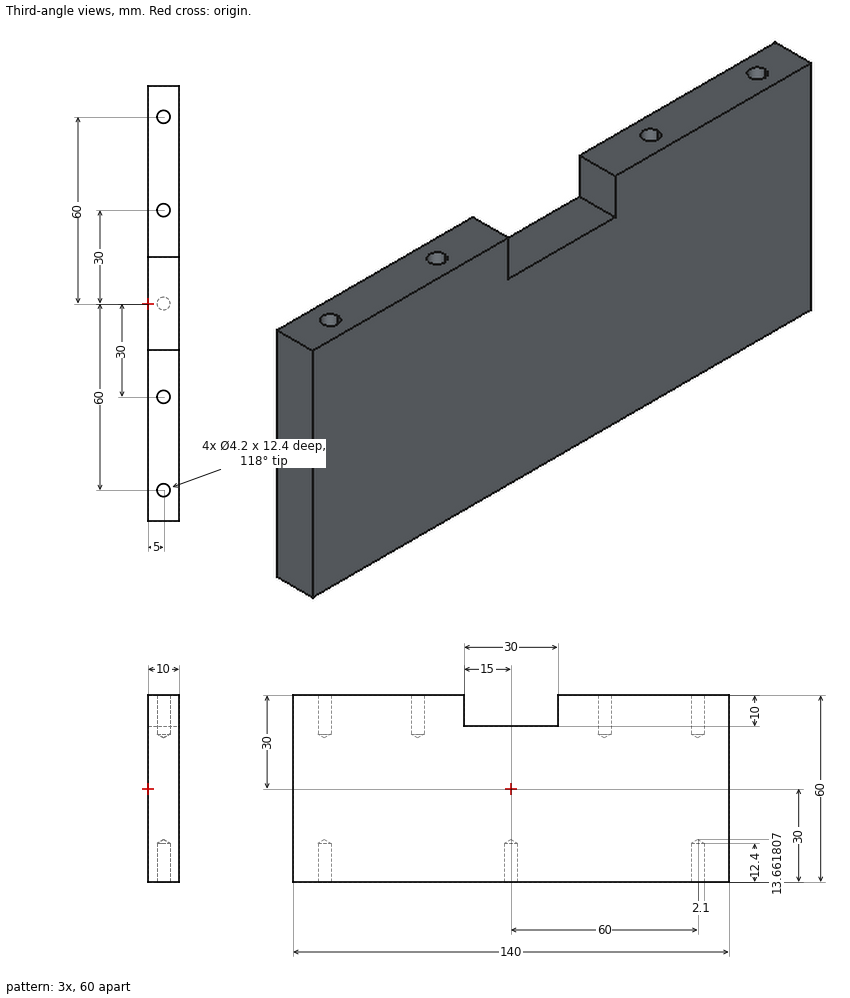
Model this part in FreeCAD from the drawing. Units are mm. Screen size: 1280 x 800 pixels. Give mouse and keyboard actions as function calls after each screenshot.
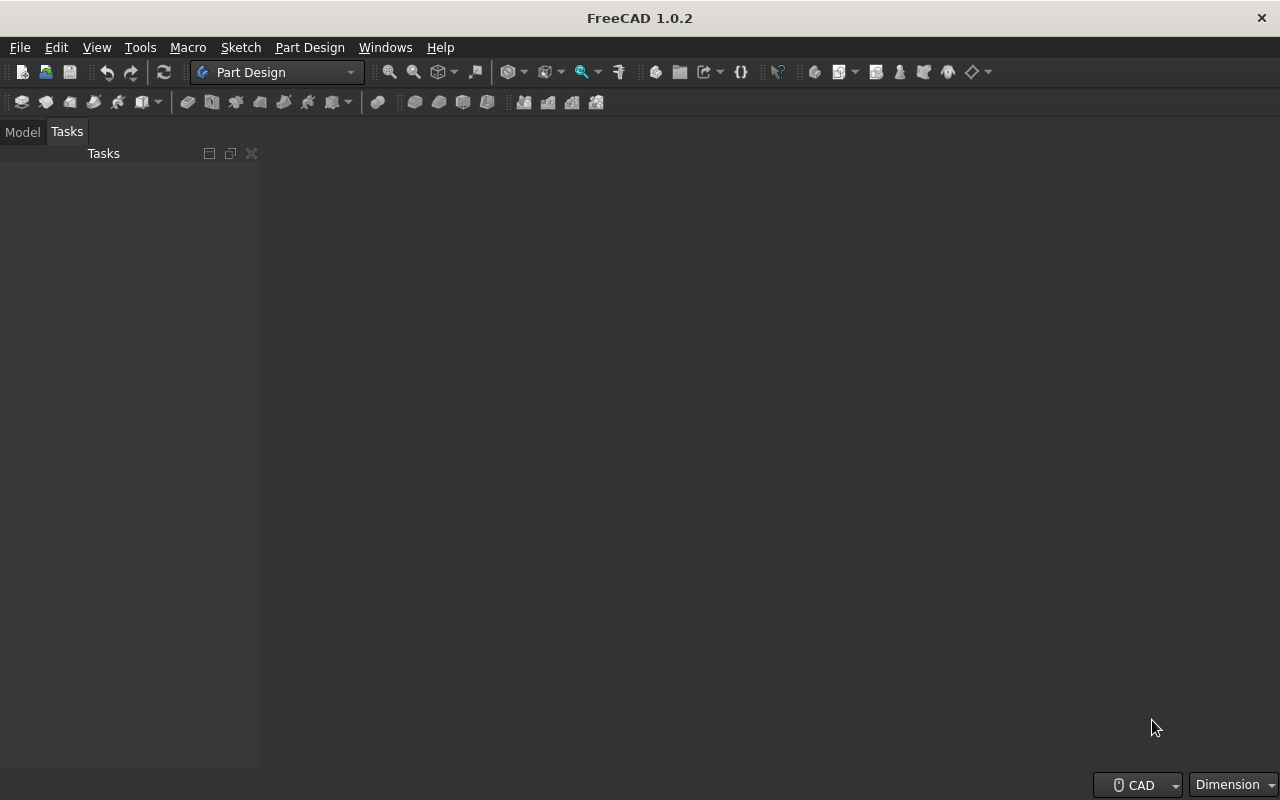
click(22, 72)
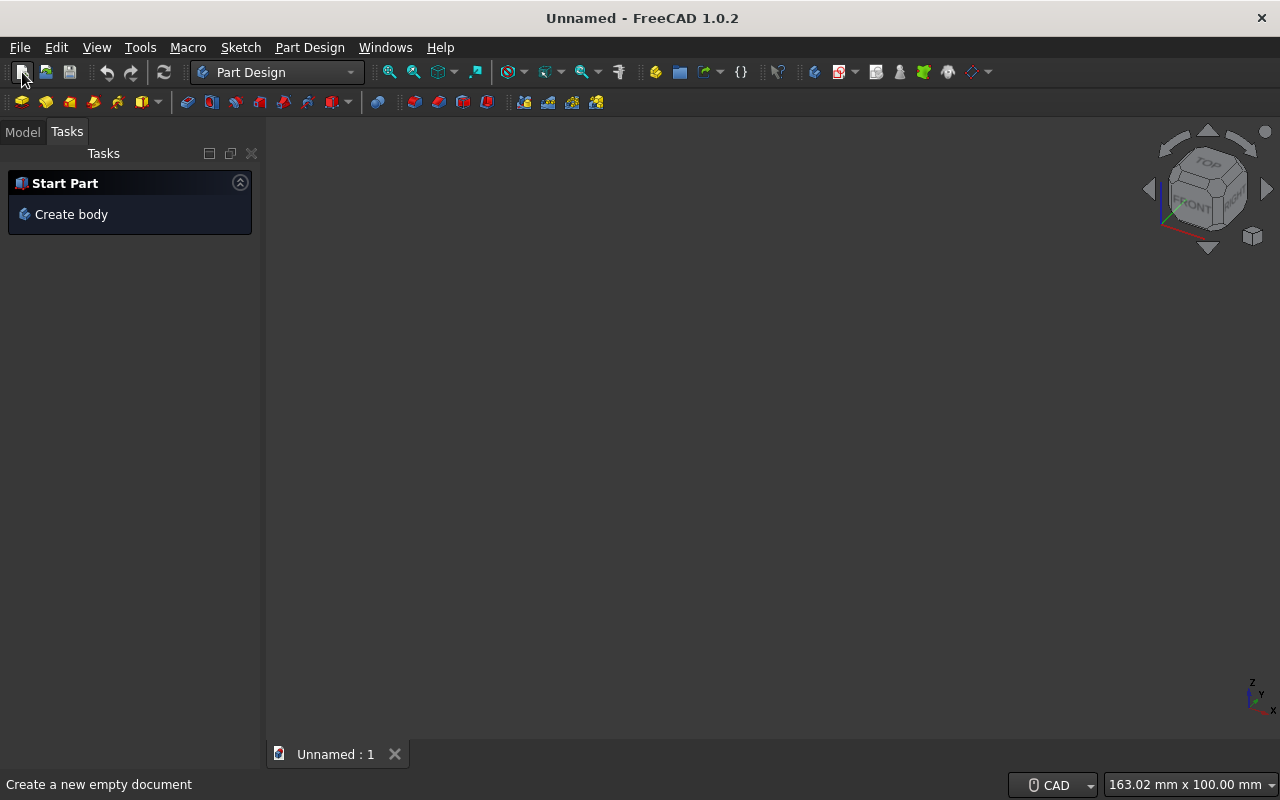
click(840, 72)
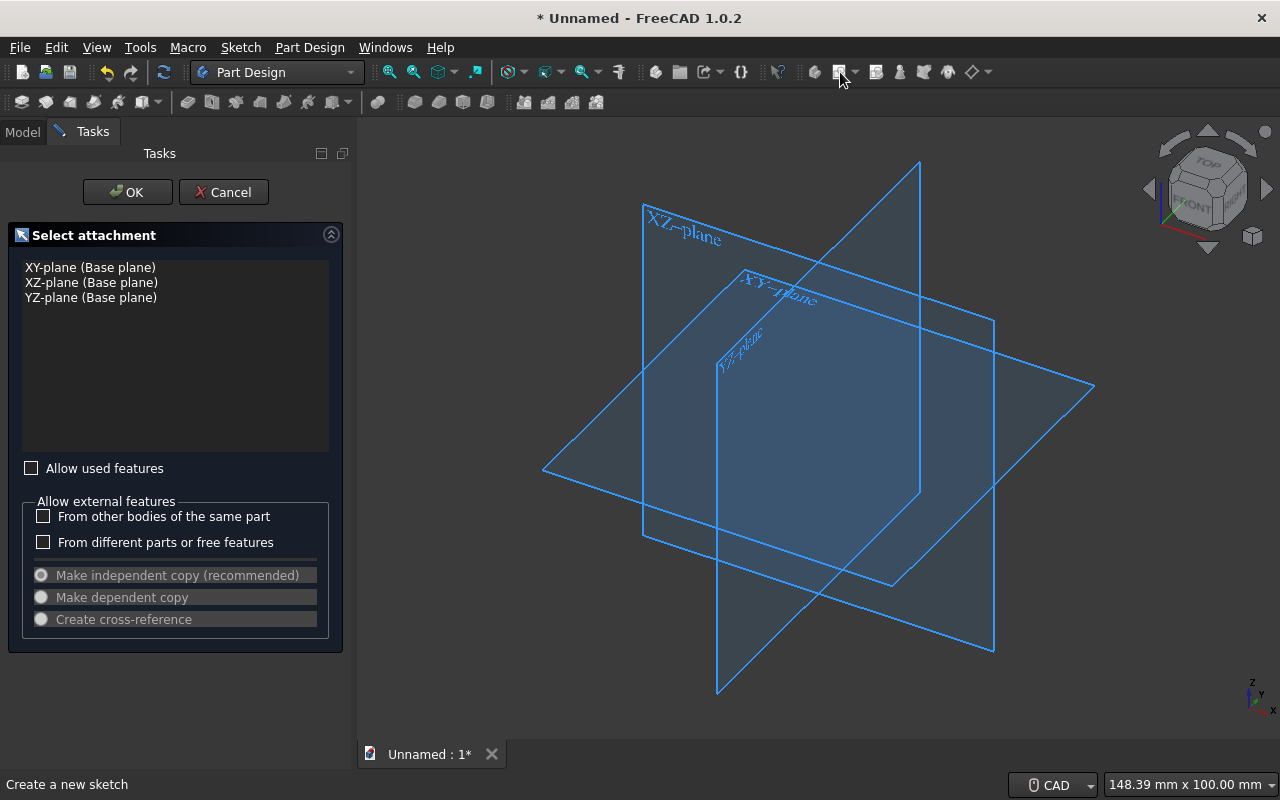
click(82, 298)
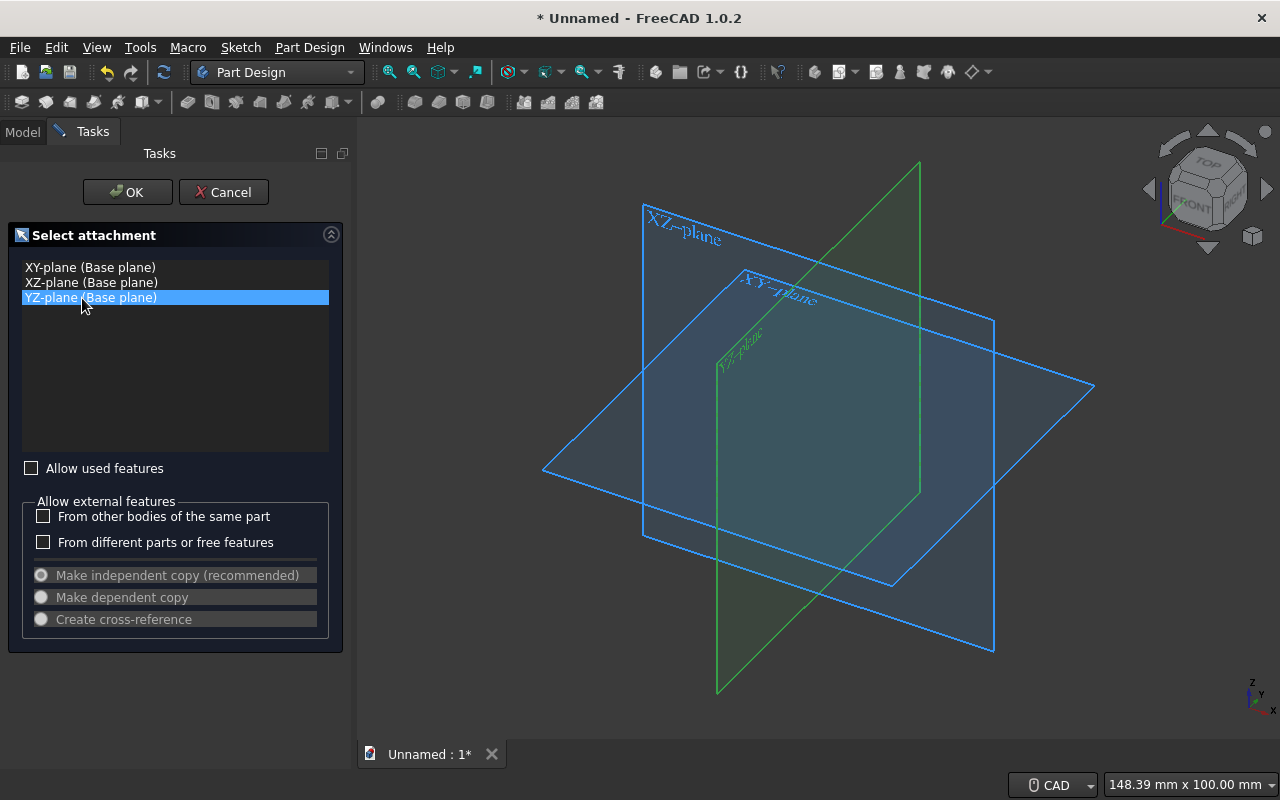
click(128, 192)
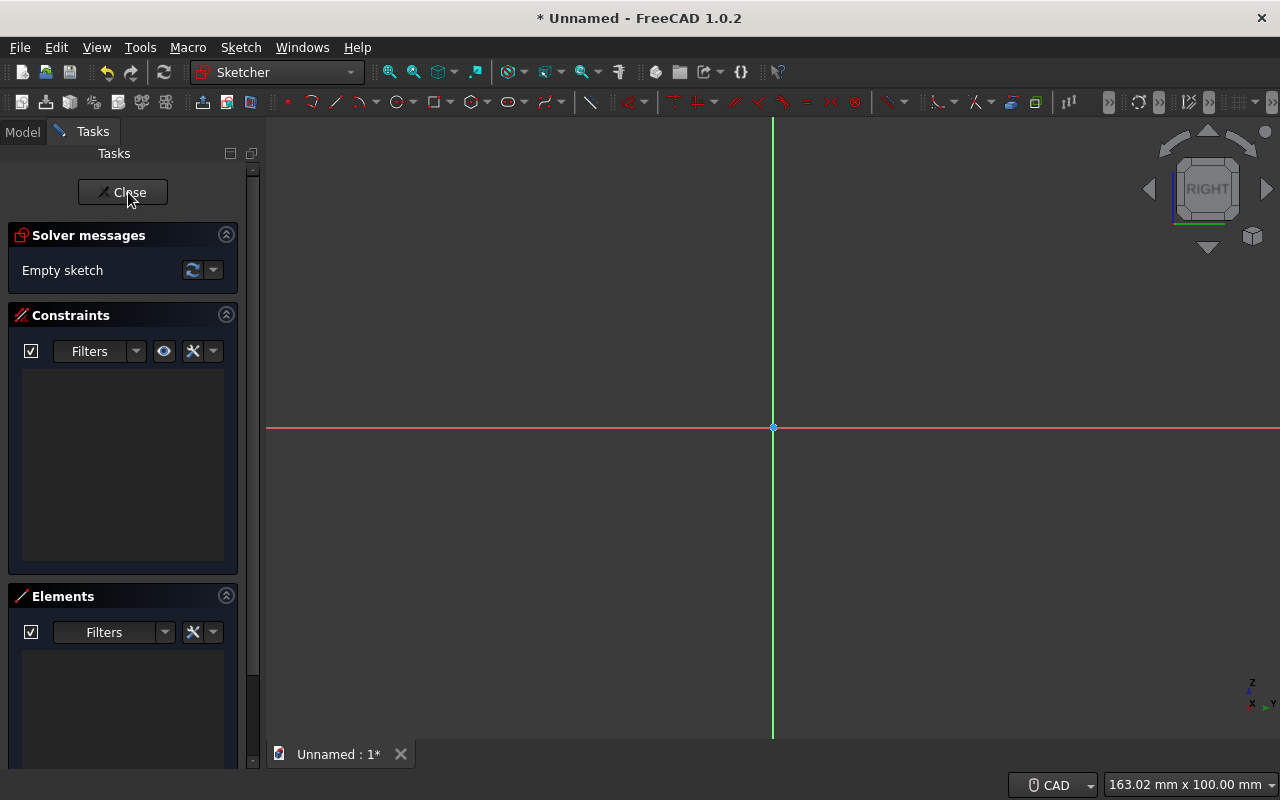
scroll(565, 428, down, 2)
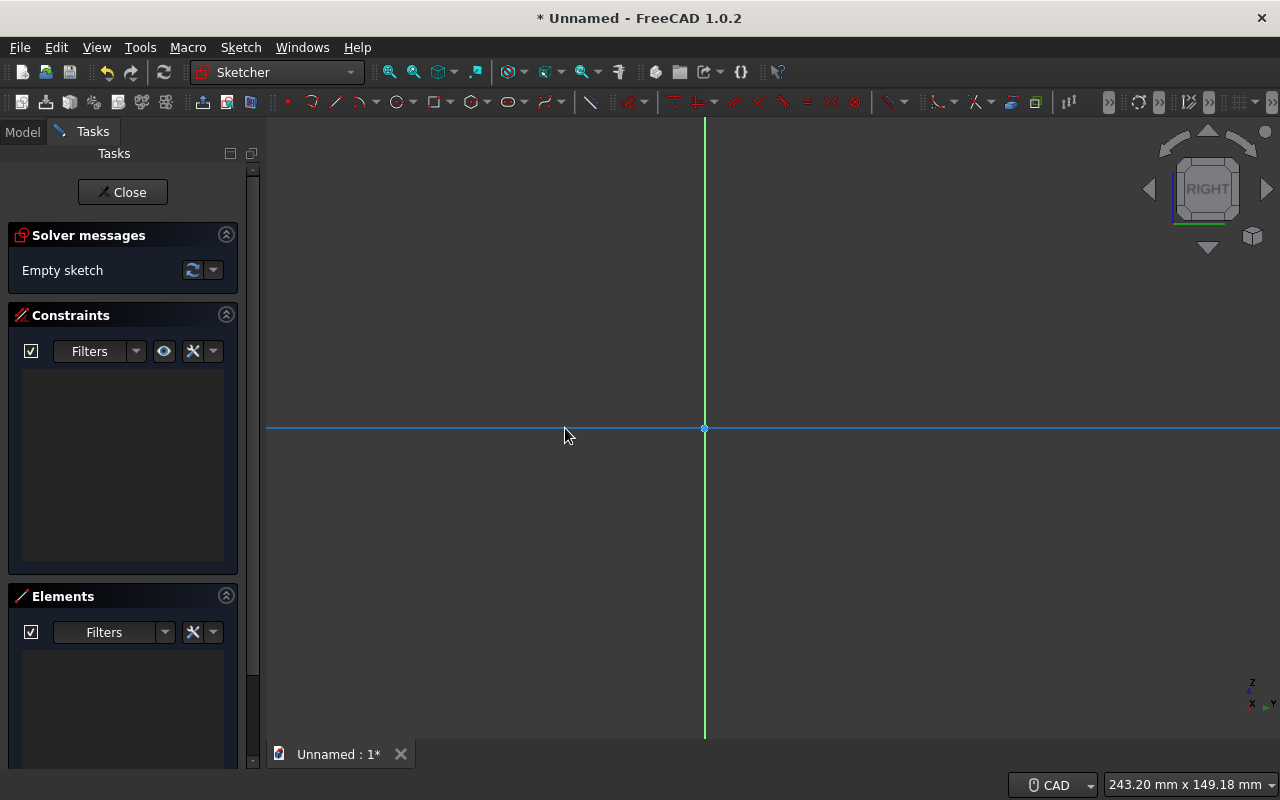
key(g)
key(v)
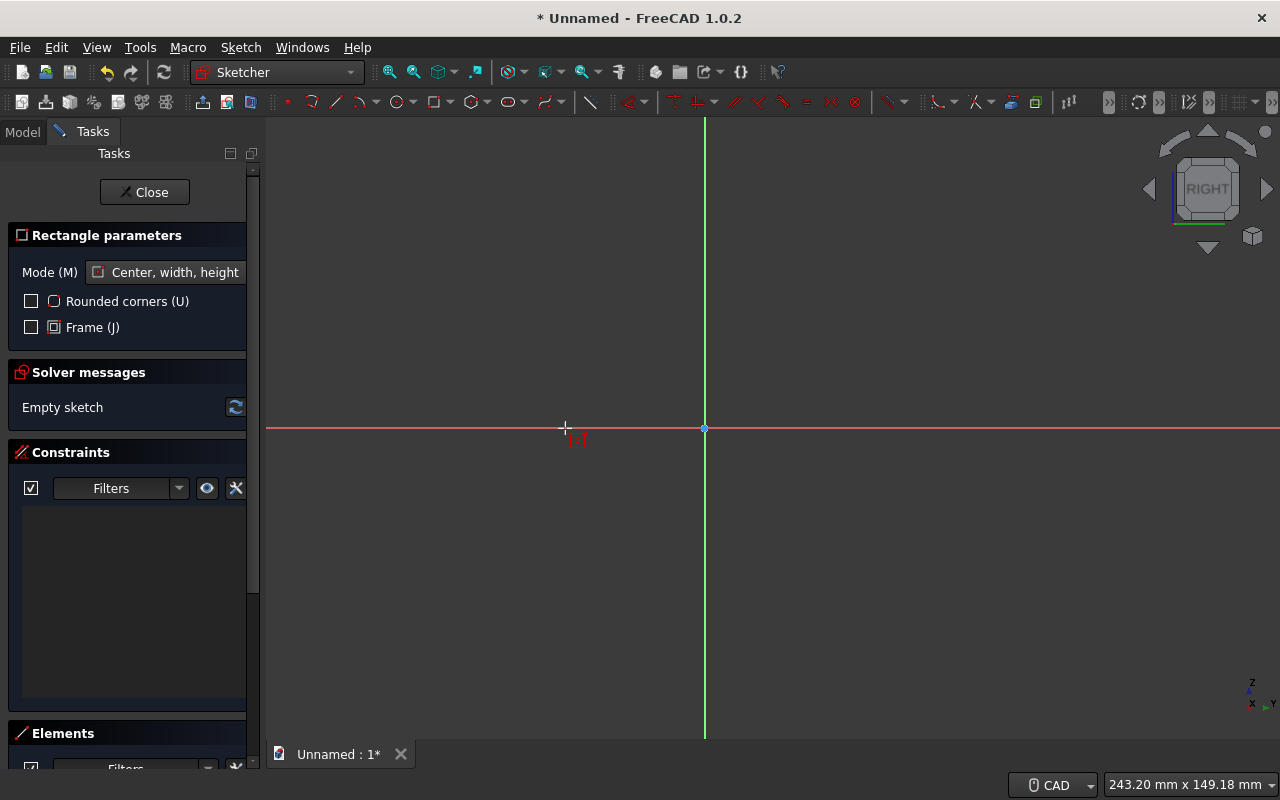
click(705, 428)
move(996, 303)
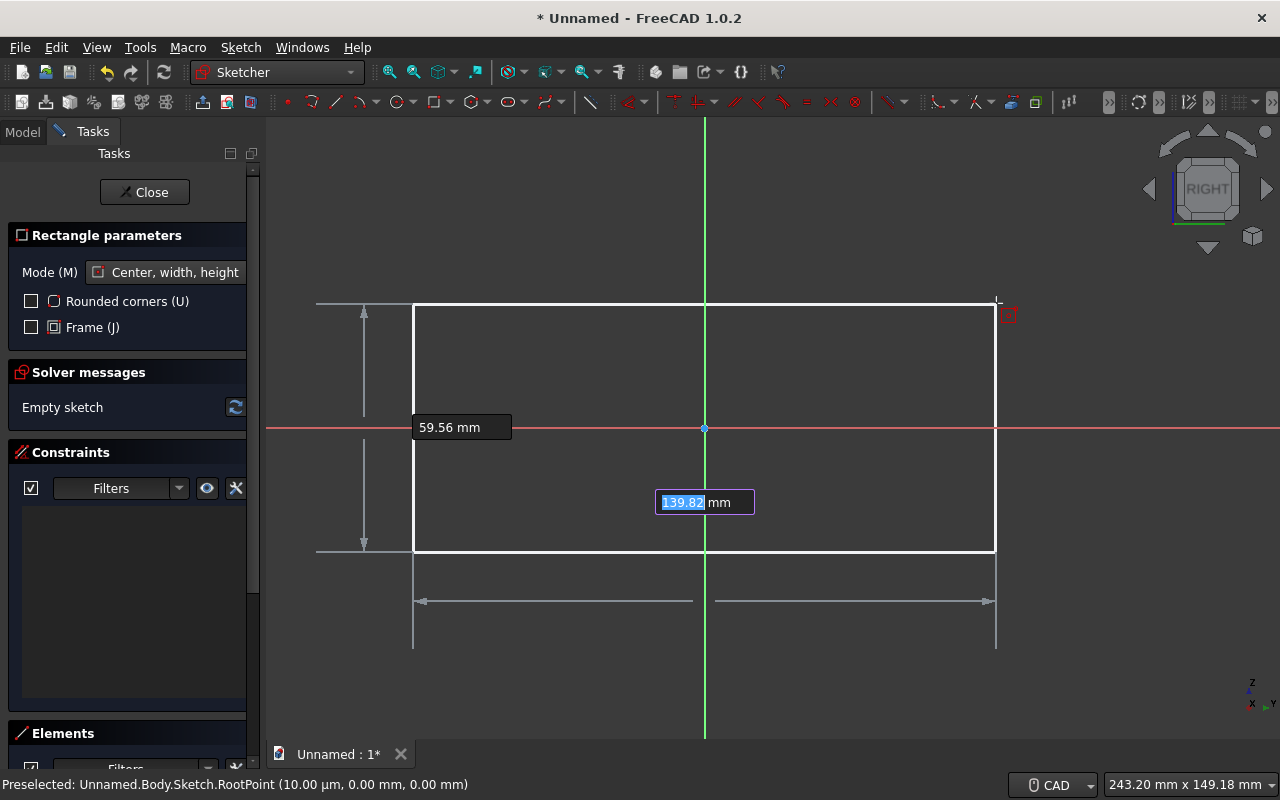
text(140)
key(Tab)
text(60)
key(Return)
key(Escape)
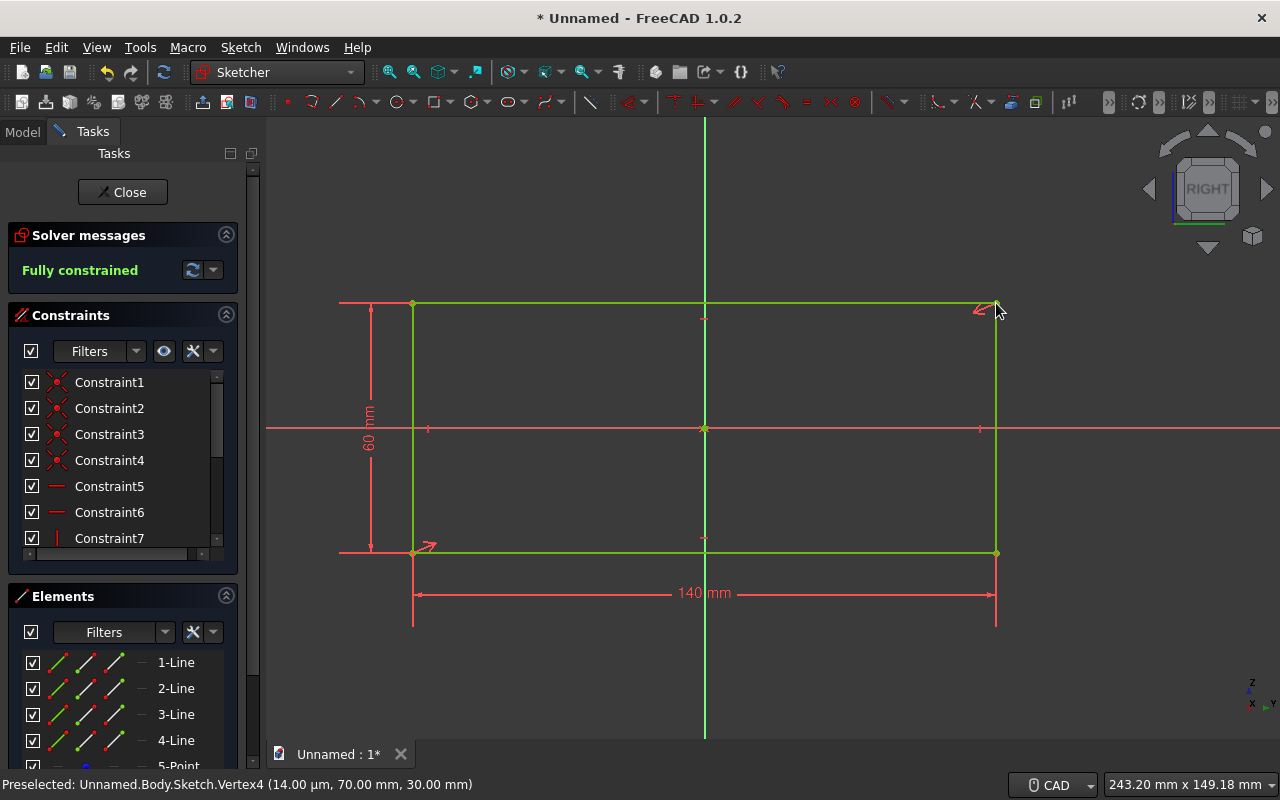
click(123, 192)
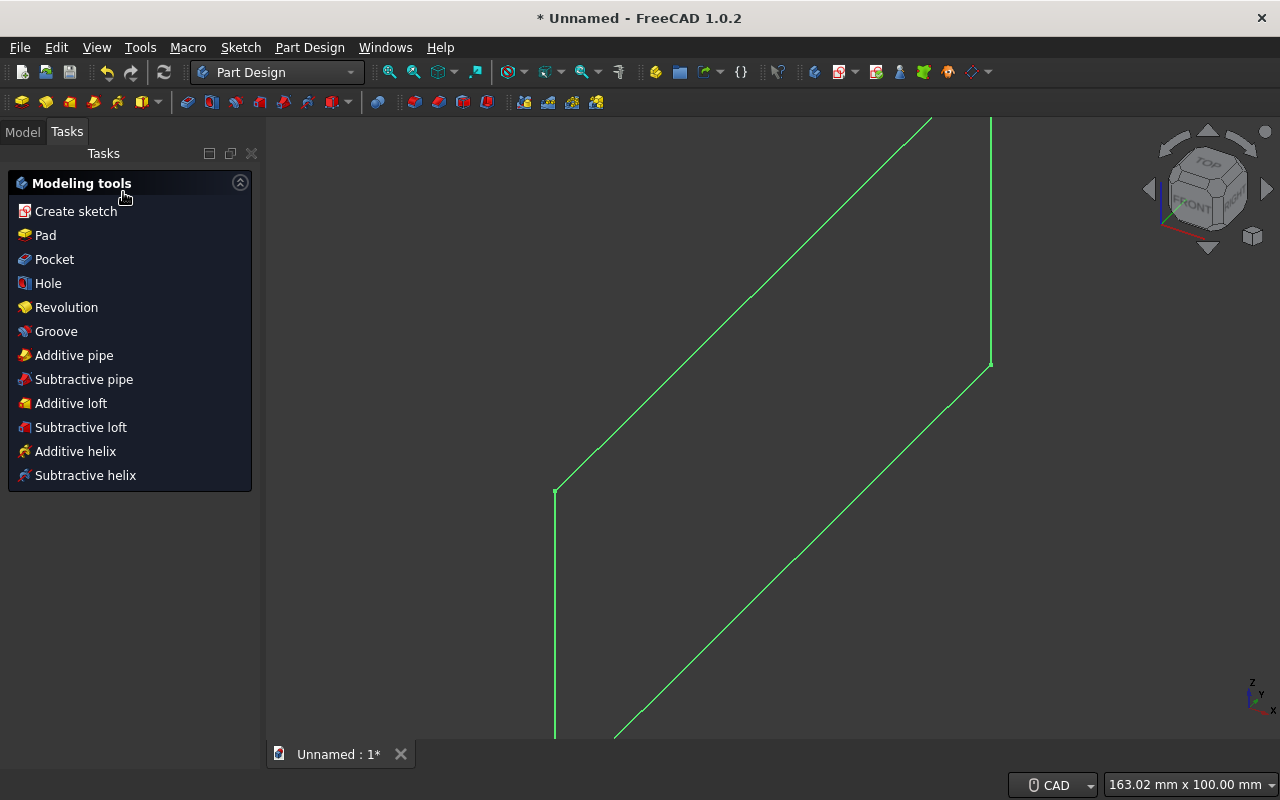
click(22, 102)